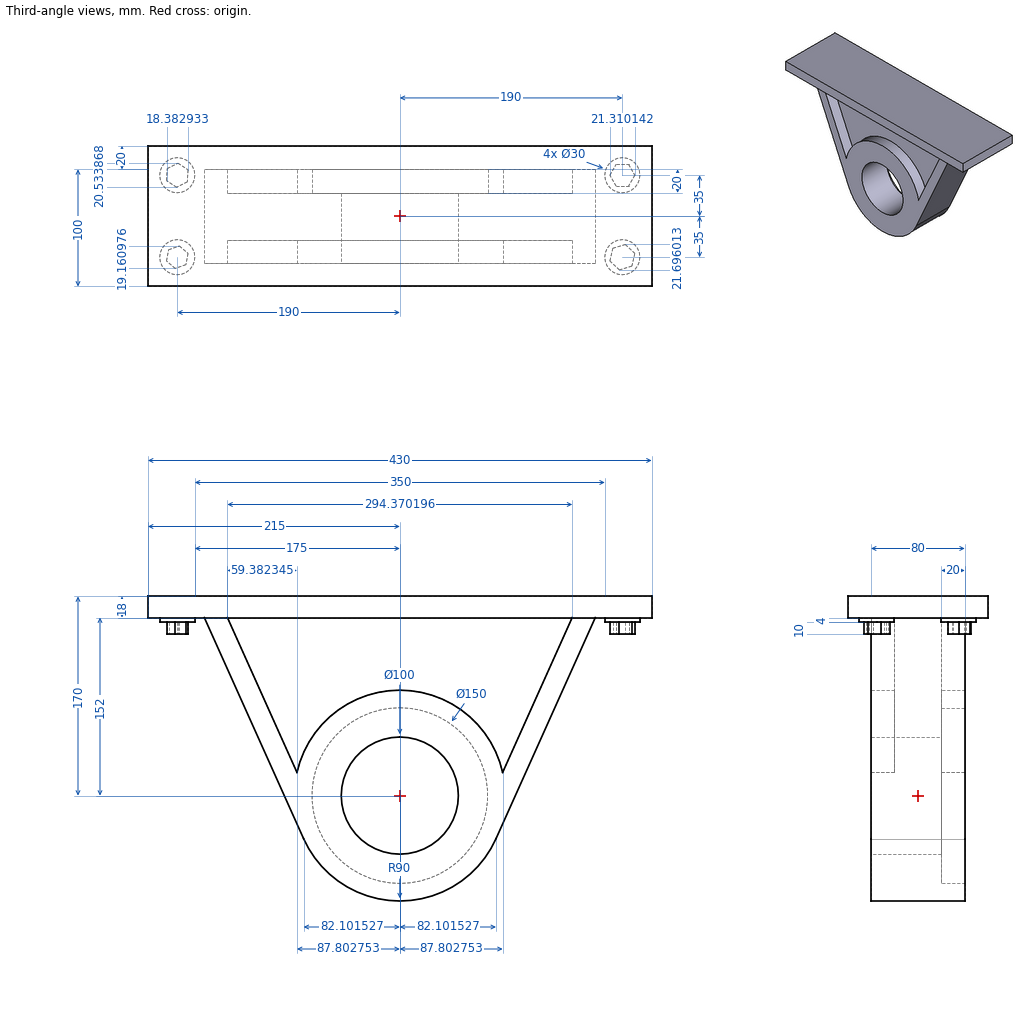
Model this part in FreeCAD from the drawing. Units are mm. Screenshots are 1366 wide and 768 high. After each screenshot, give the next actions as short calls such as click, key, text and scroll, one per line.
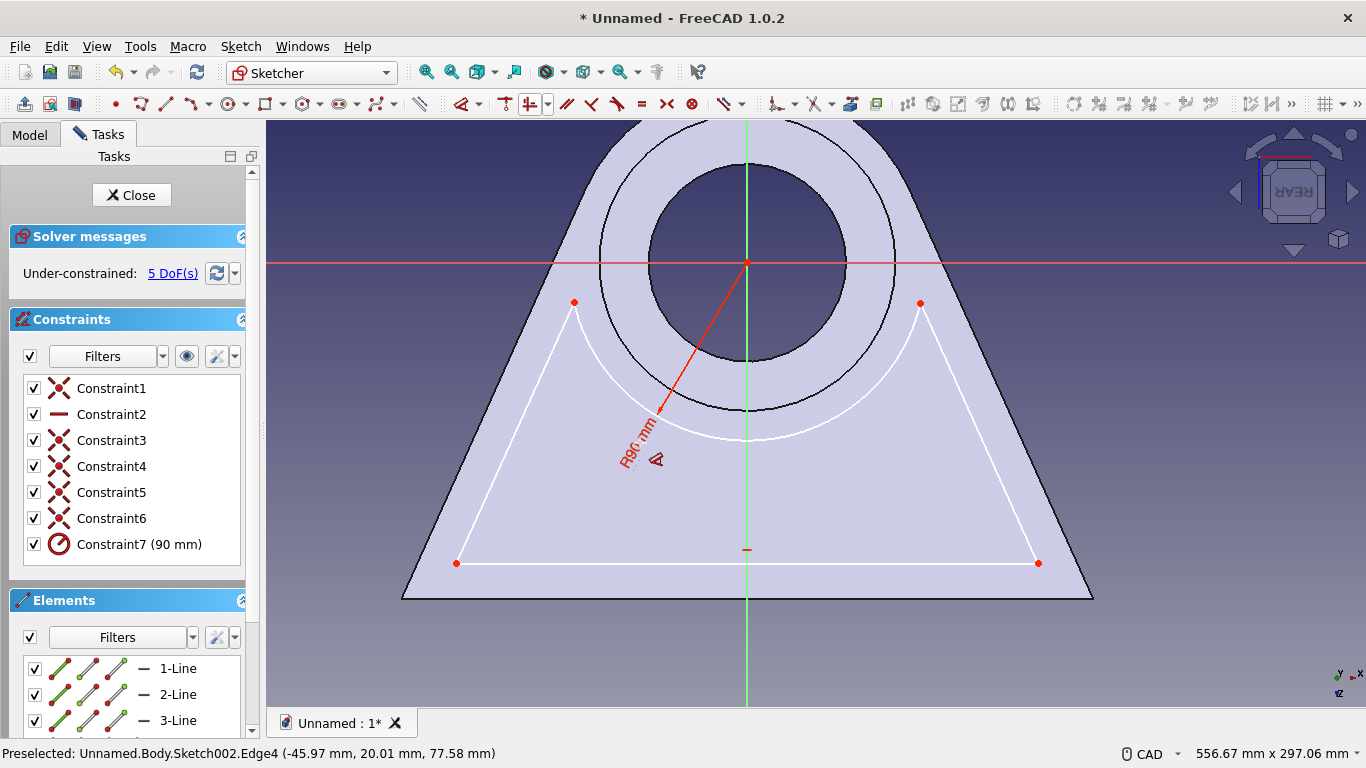
click(456, 564)
click(422, 413)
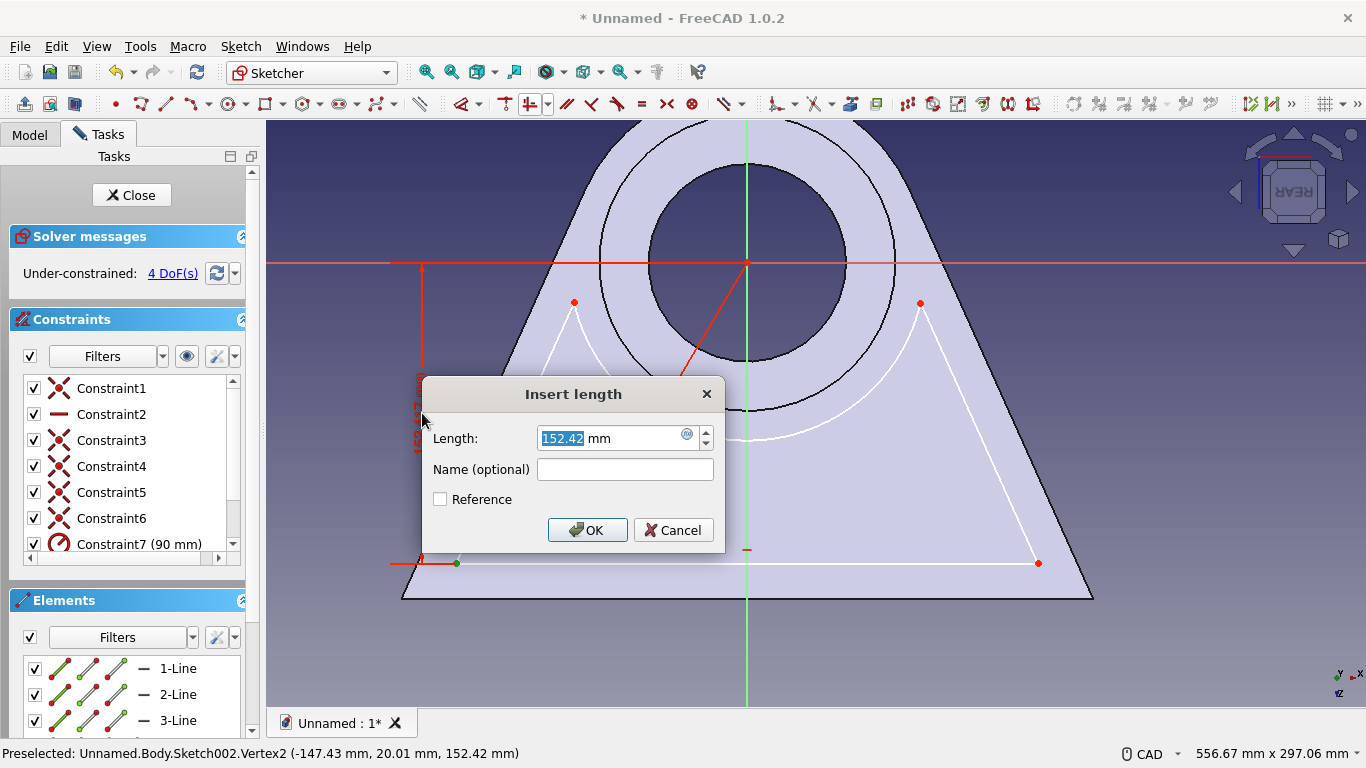
text(152)
key(Return)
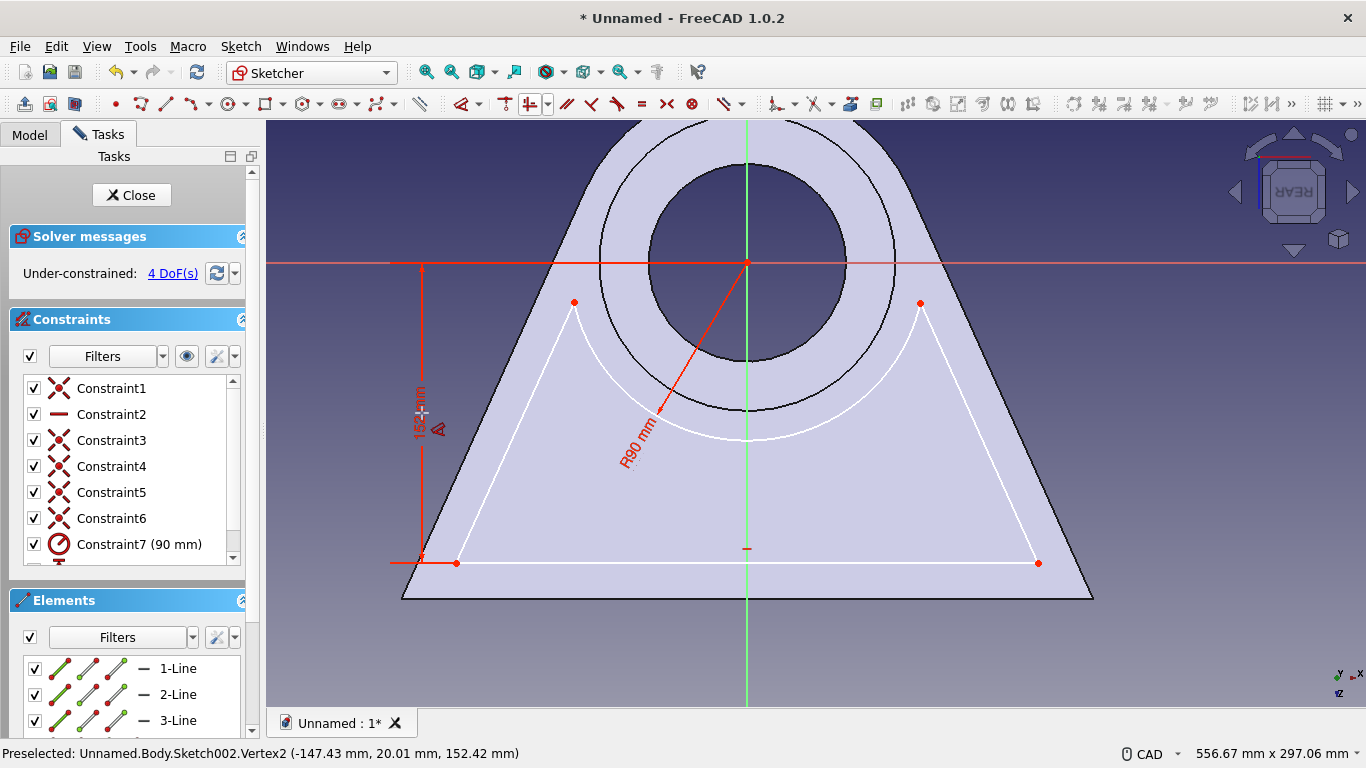
click(631, 563)
click(613, 597)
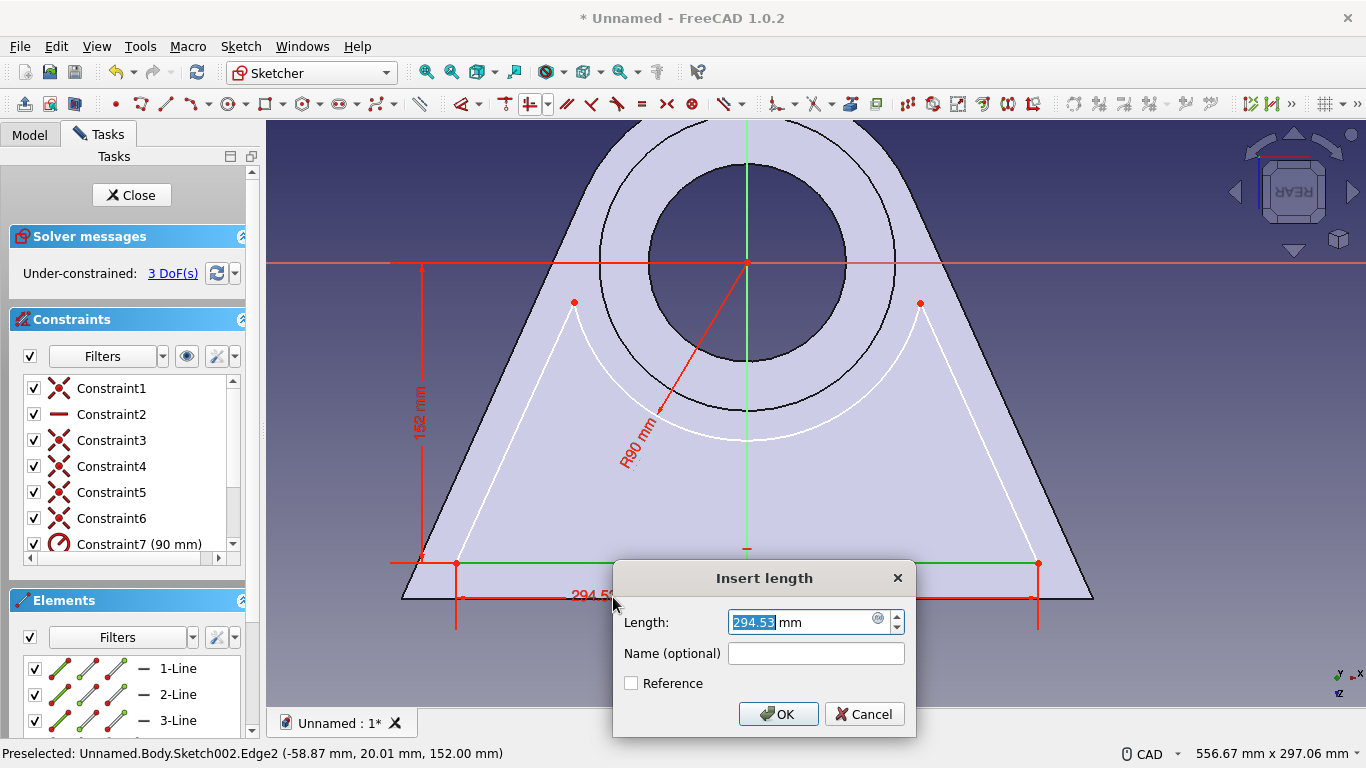
text(294.370196)
key(Return)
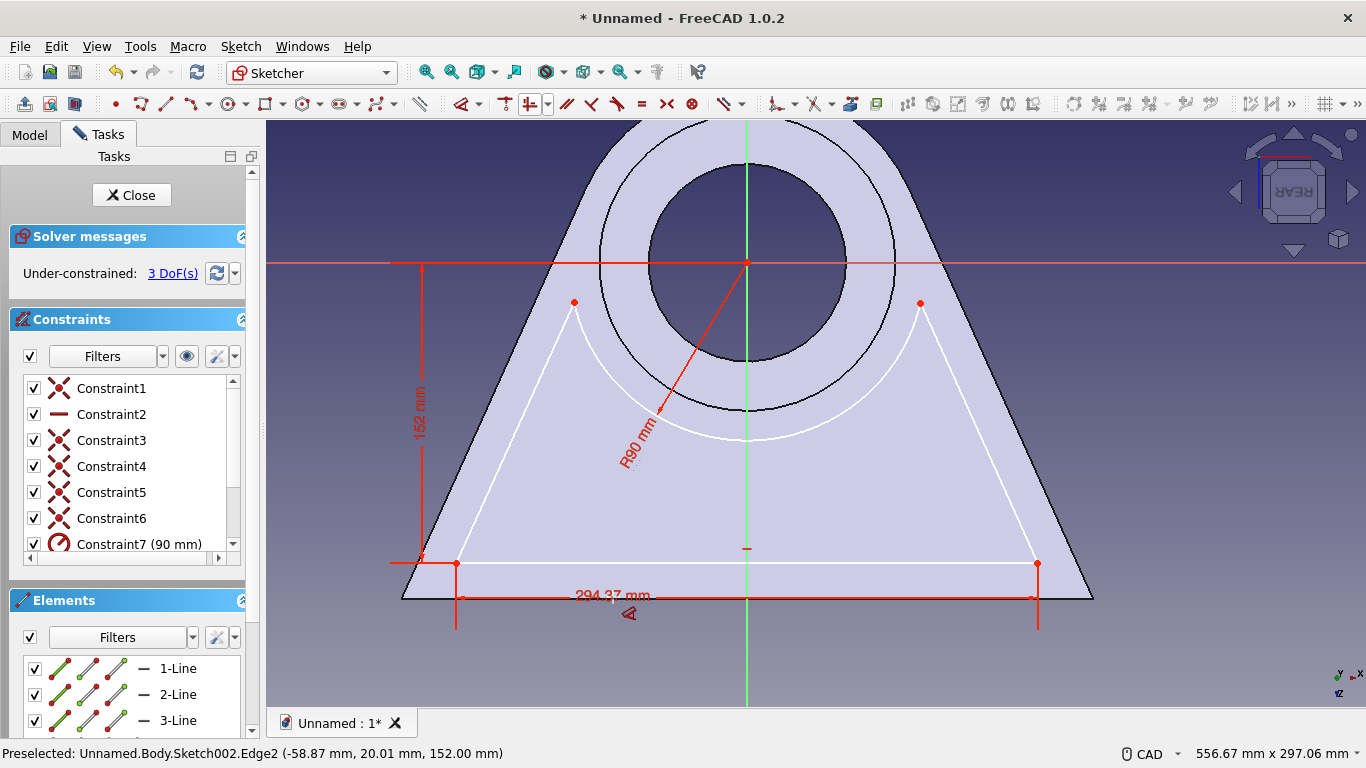
click(574, 303)
click(661, 229)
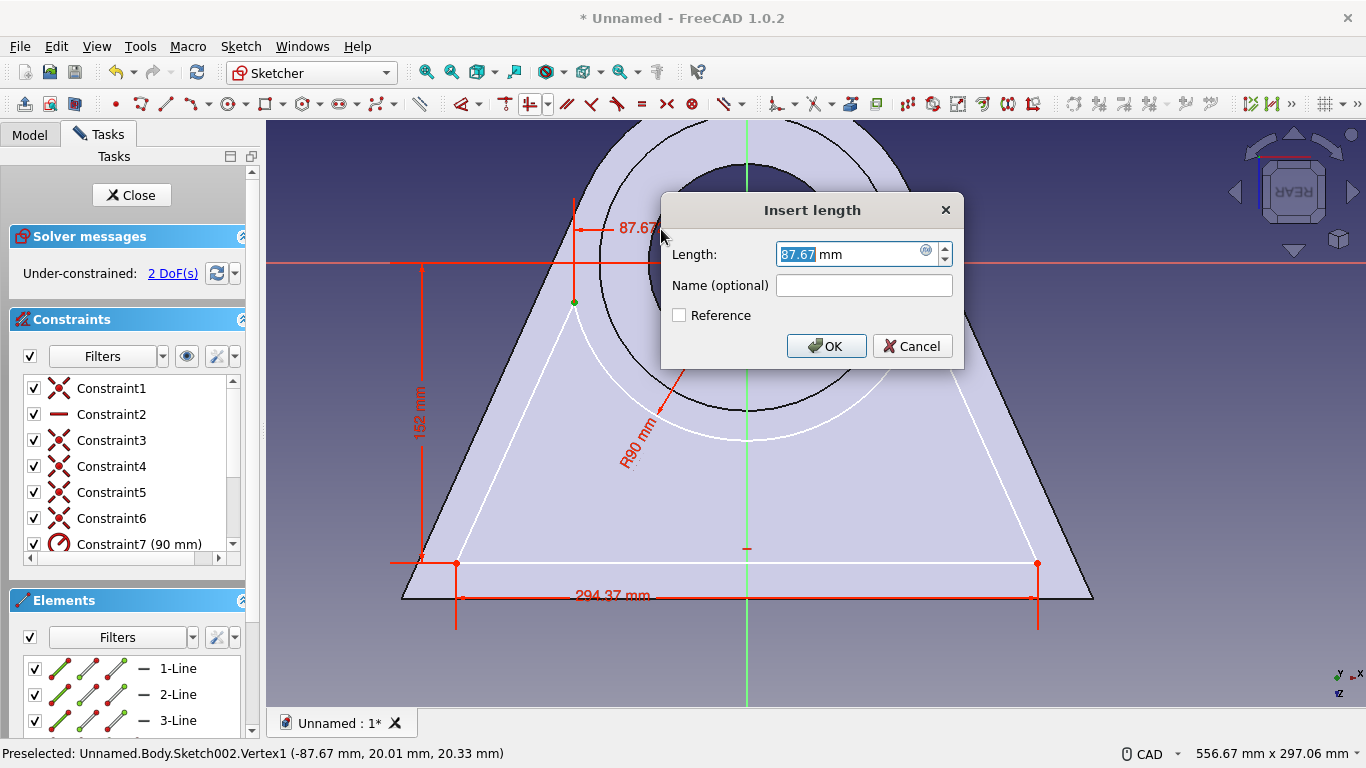
text(87.802753)
key(Return)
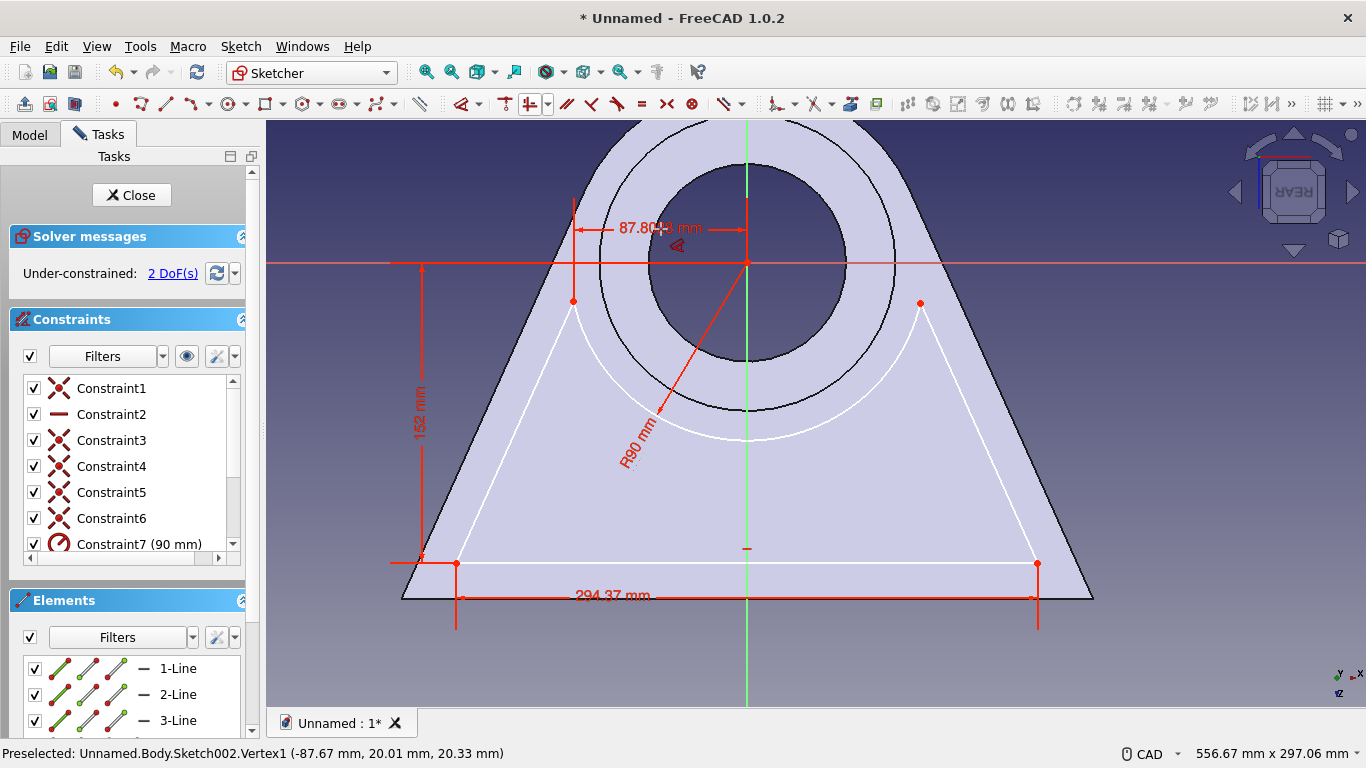
click(921, 303)
click(834, 229)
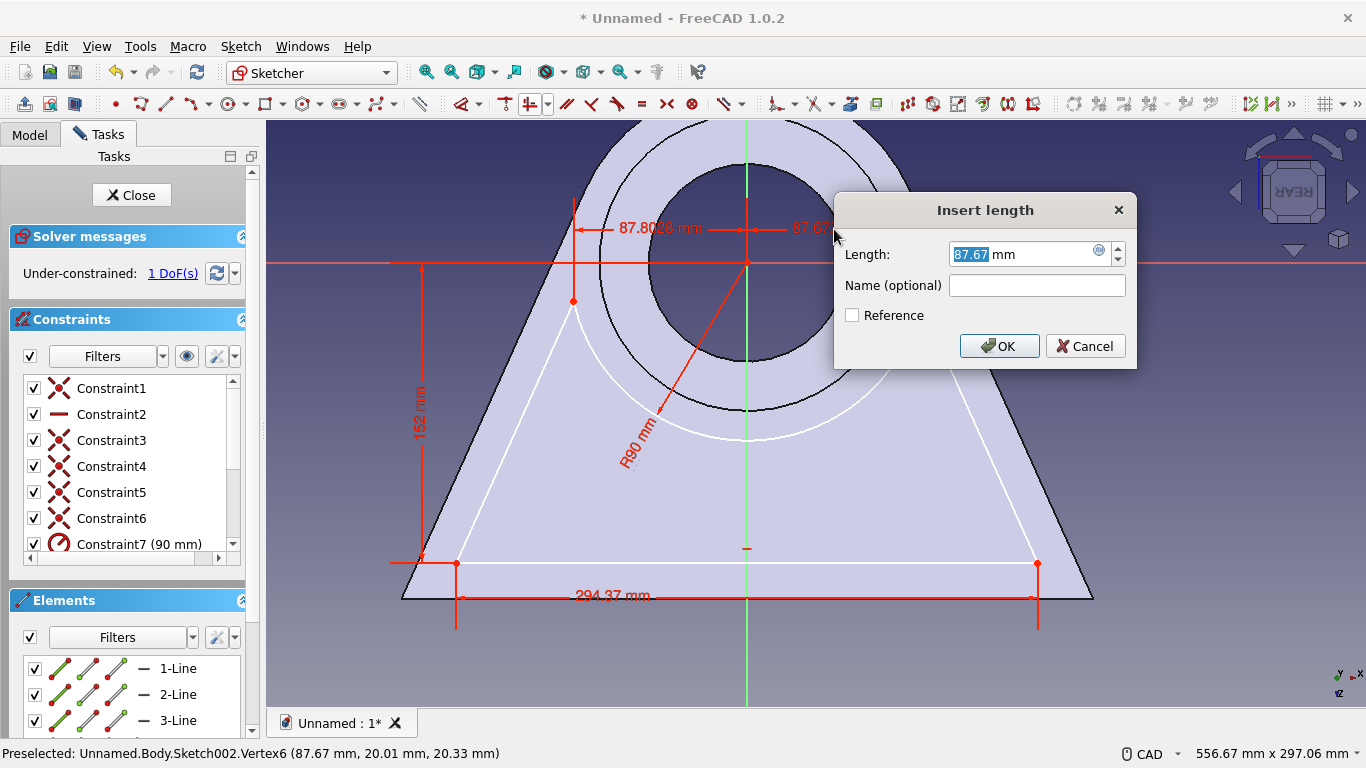
text(87.802753)
key(Return)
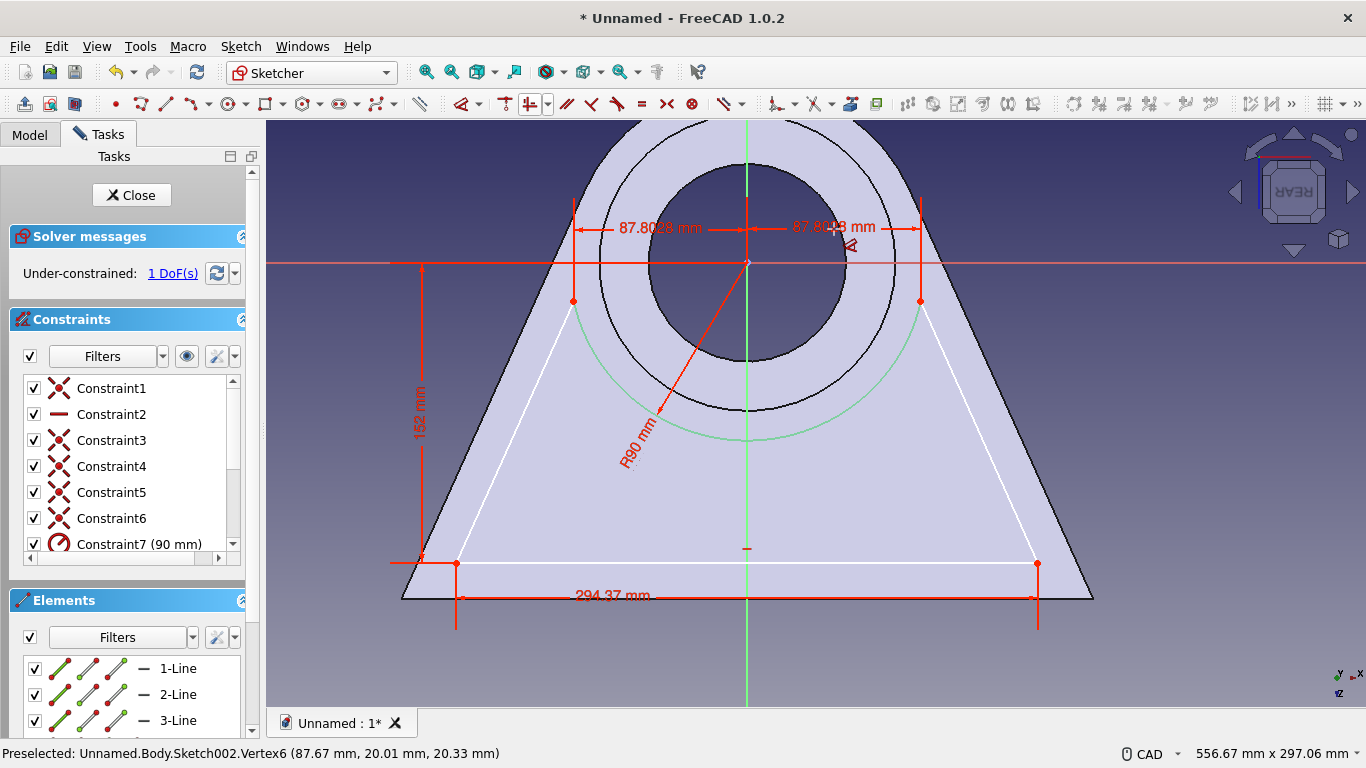
click(539, 380)
click(515, 597)